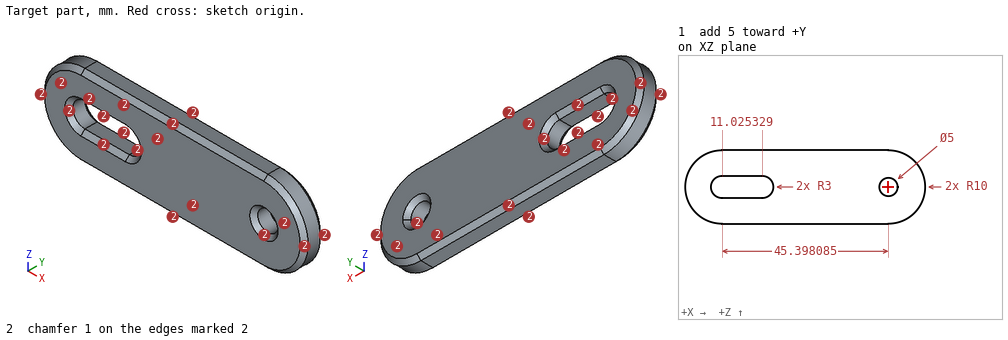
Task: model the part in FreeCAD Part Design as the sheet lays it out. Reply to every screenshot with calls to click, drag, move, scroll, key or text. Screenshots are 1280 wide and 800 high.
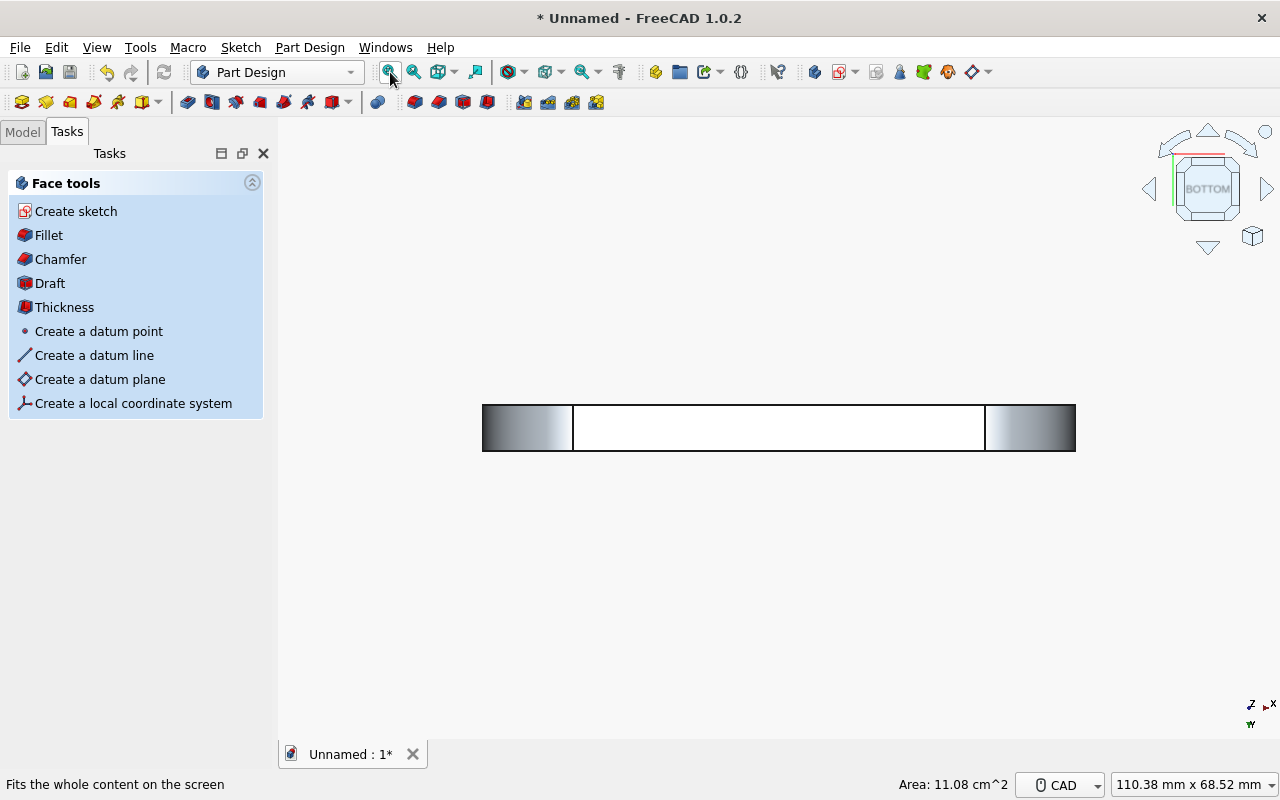
key(4)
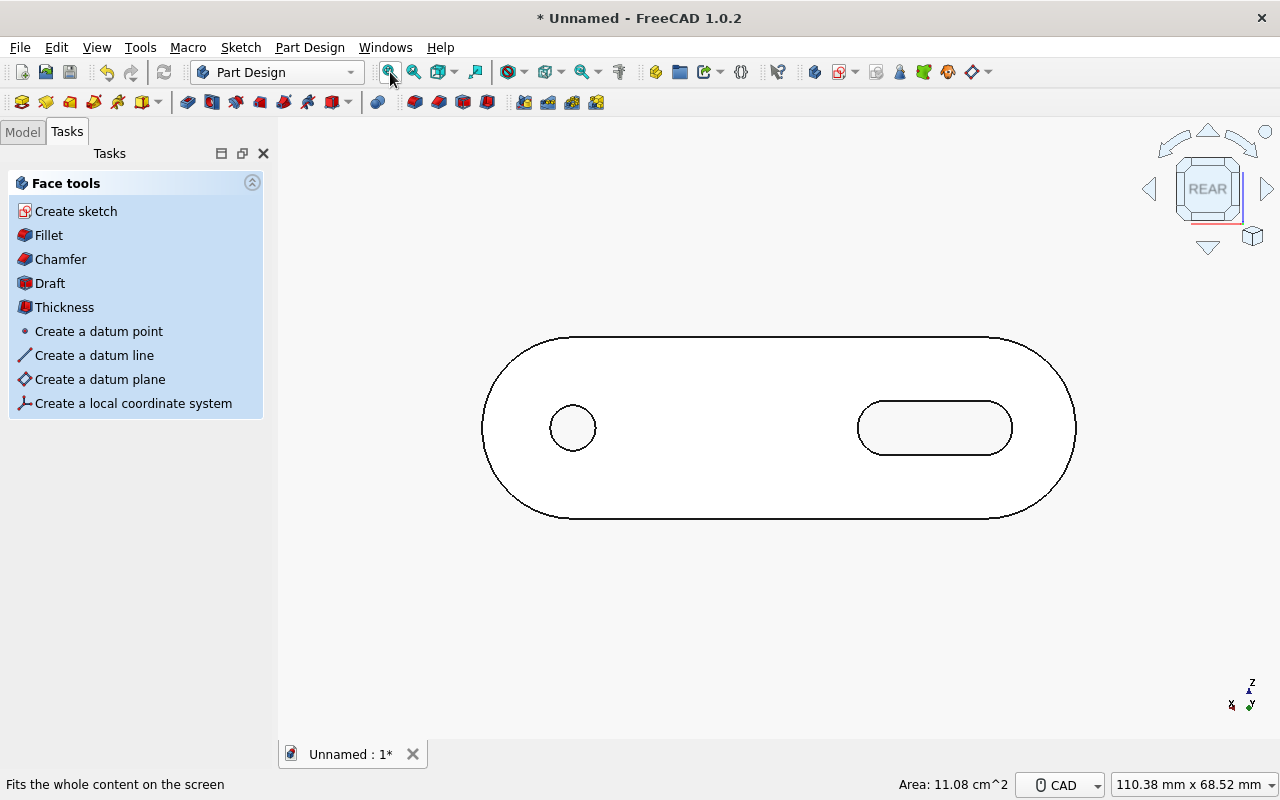
click(694, 427, ctrl)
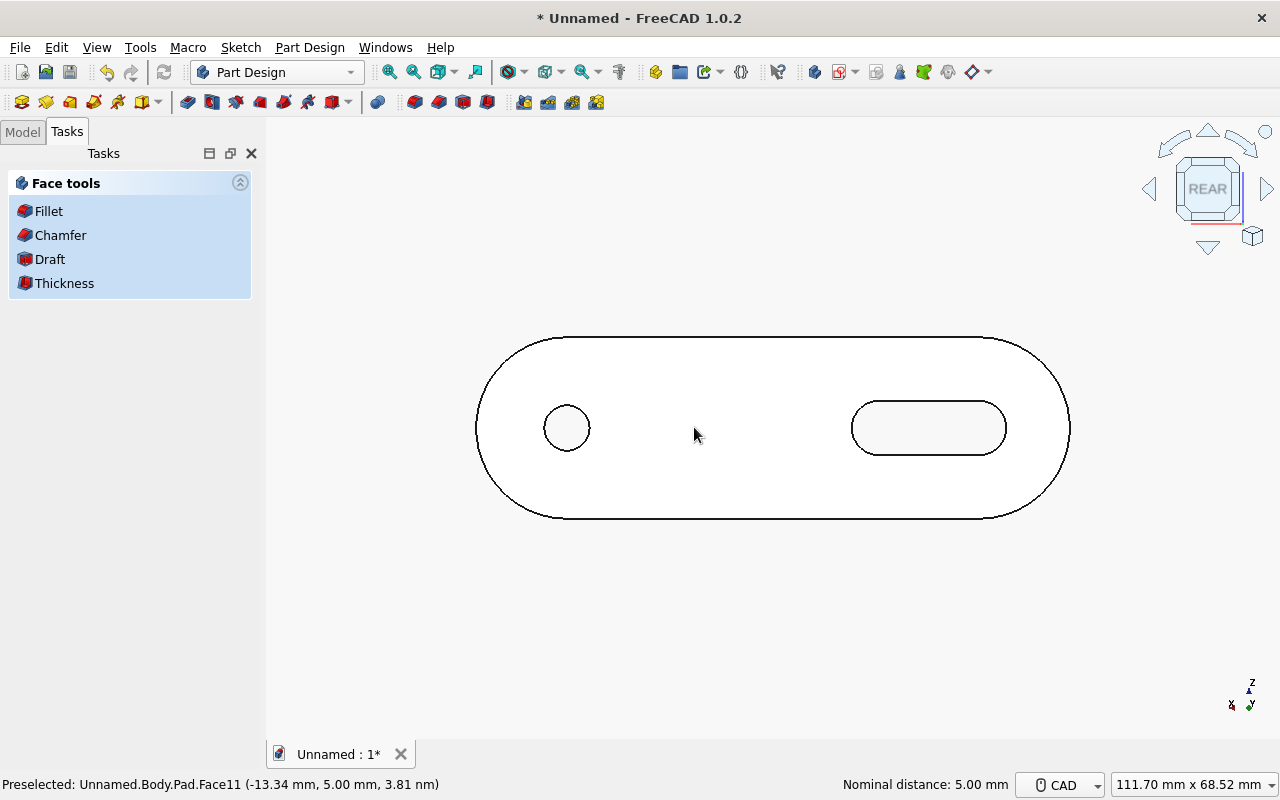
click(440, 102)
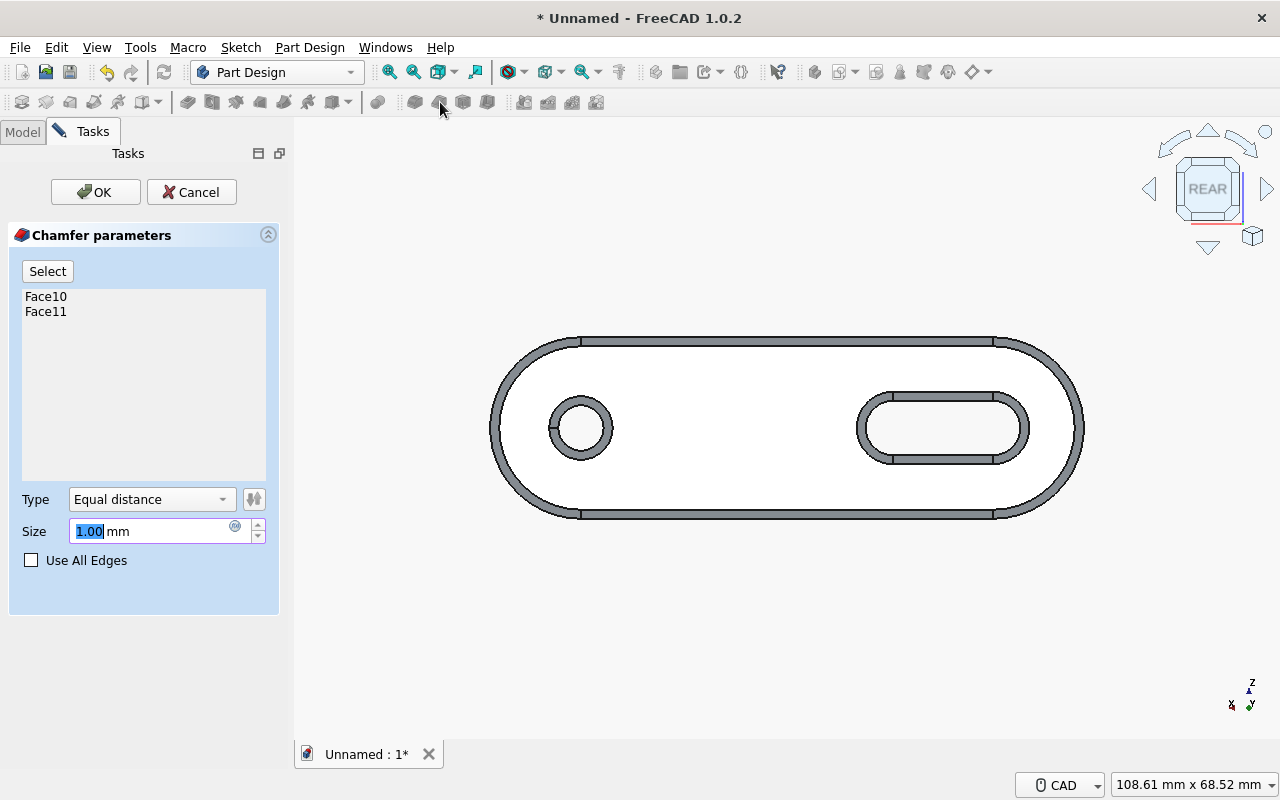
text(1)
key(Tab)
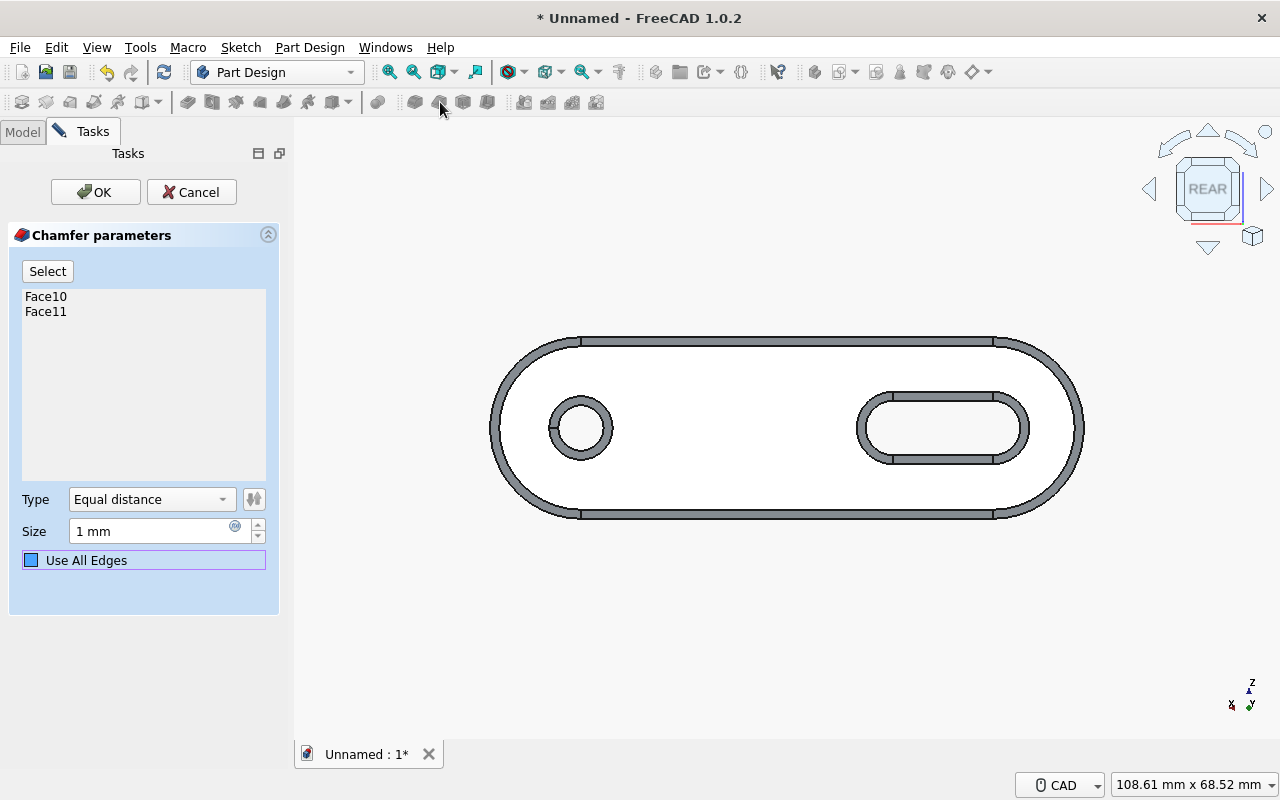
click(96, 192)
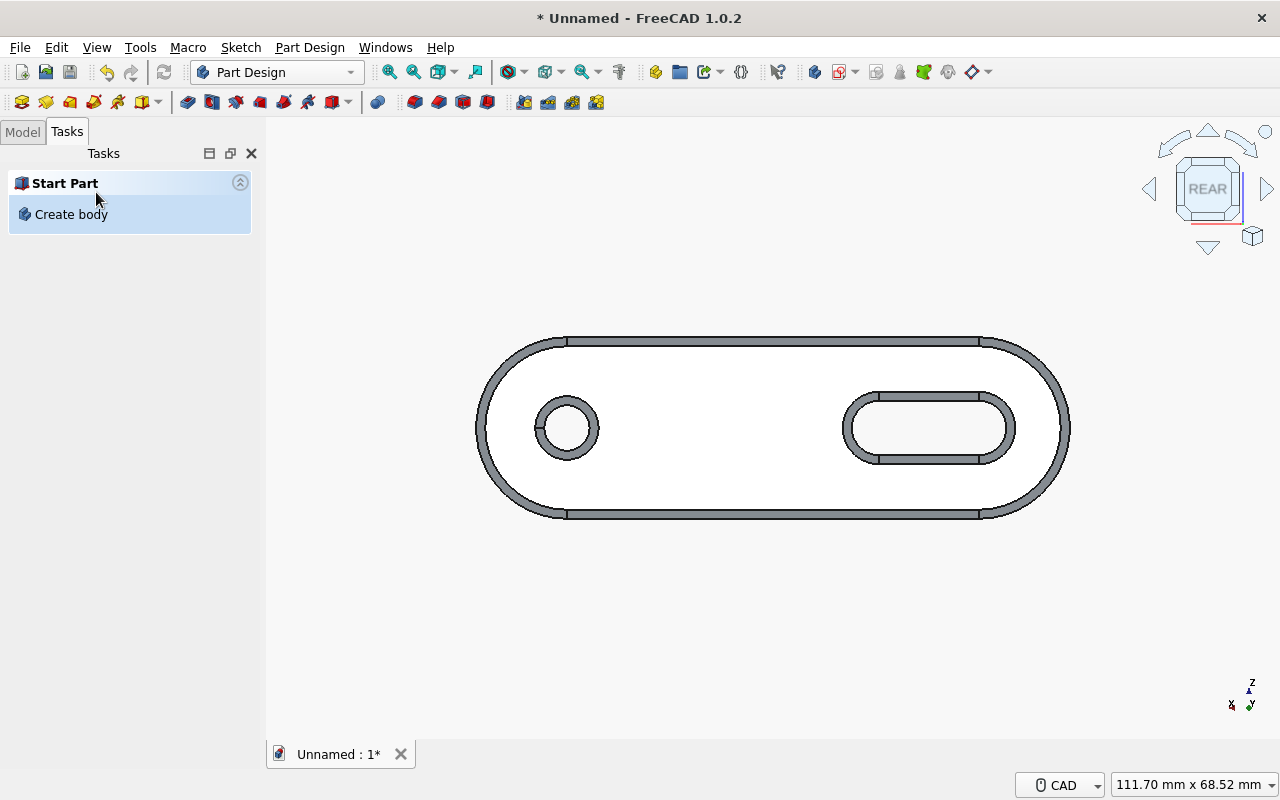
key(0)